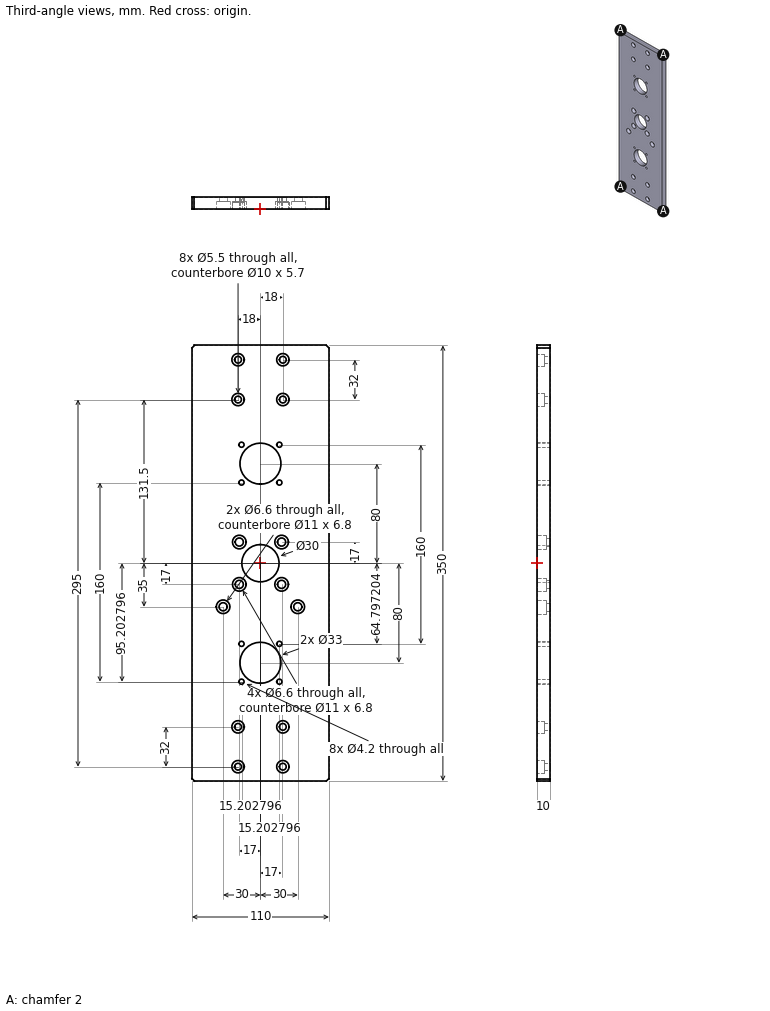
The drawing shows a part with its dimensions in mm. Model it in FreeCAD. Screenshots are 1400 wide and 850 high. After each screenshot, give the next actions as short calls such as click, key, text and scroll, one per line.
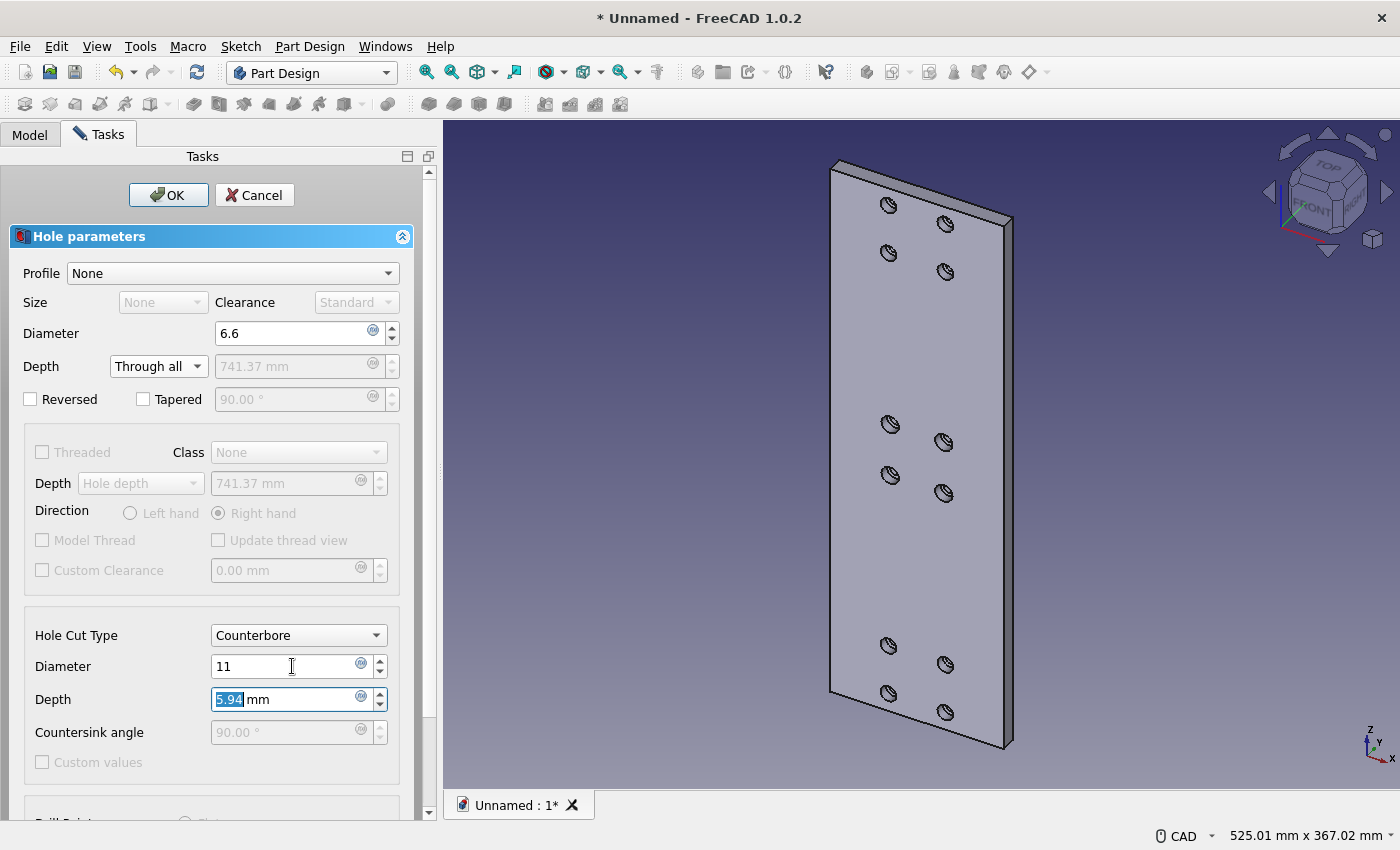
text(6.8)
key(Tab)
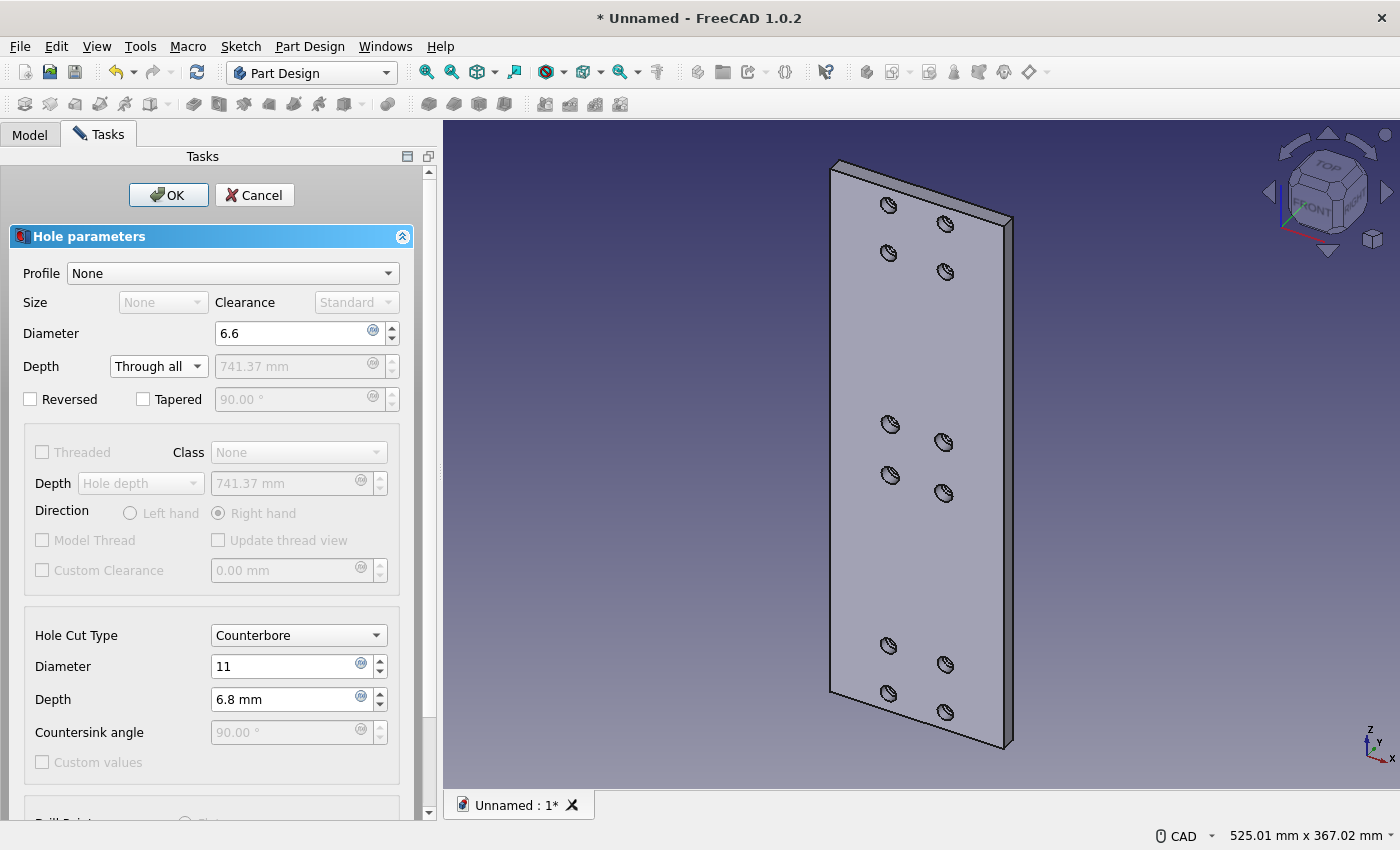
click(169, 195)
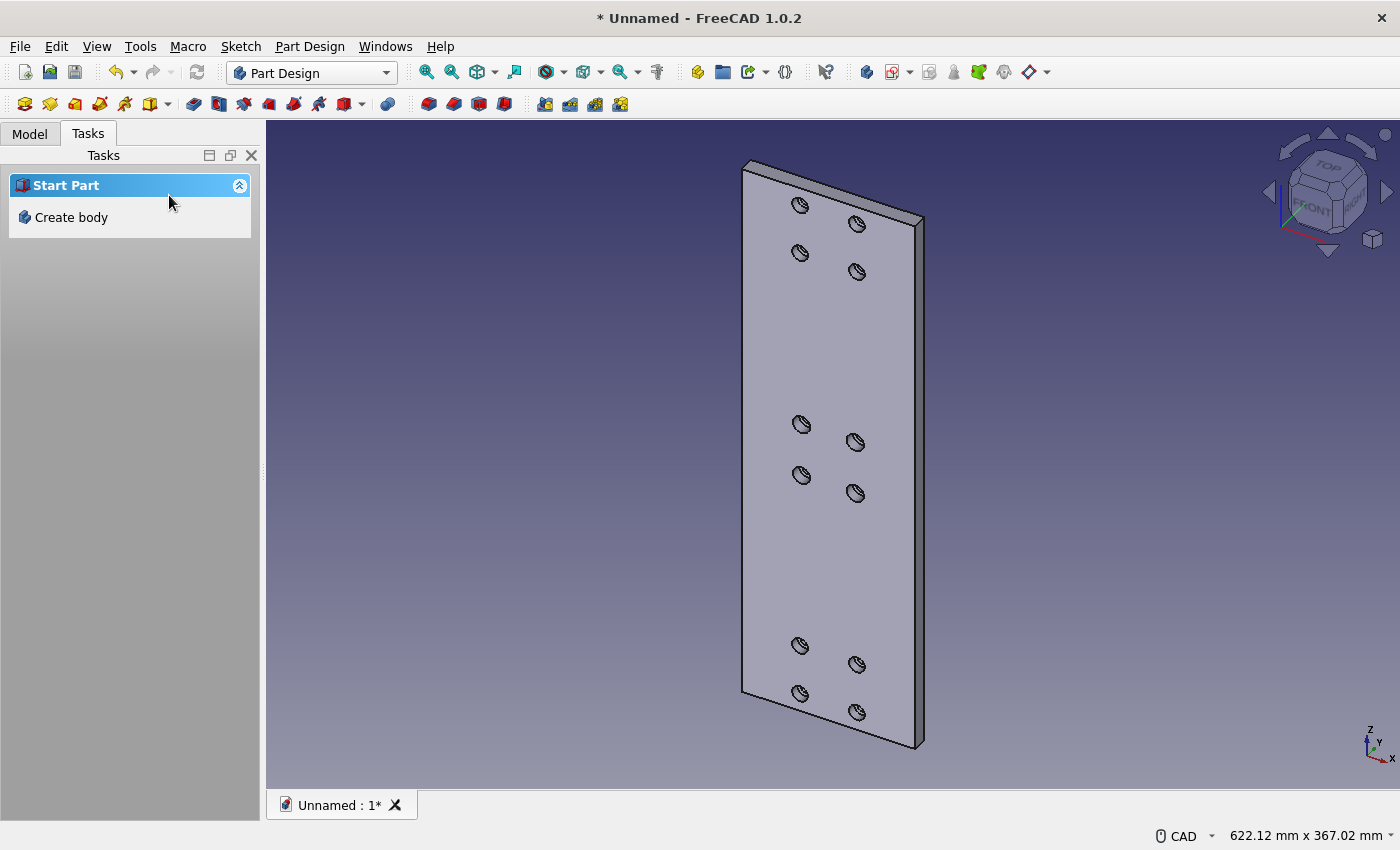
click(920, 221)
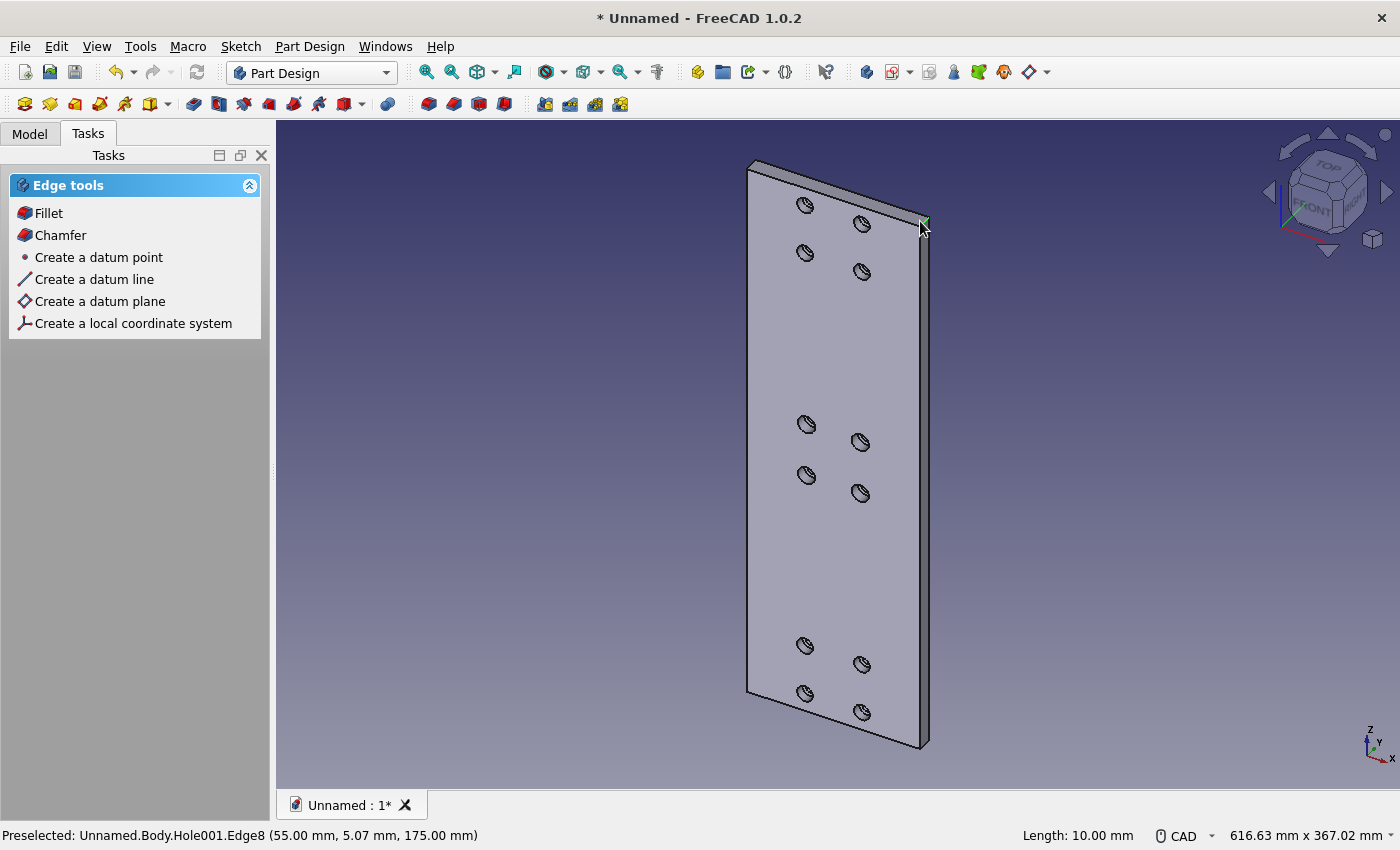
scroll(751, 163, up, 4)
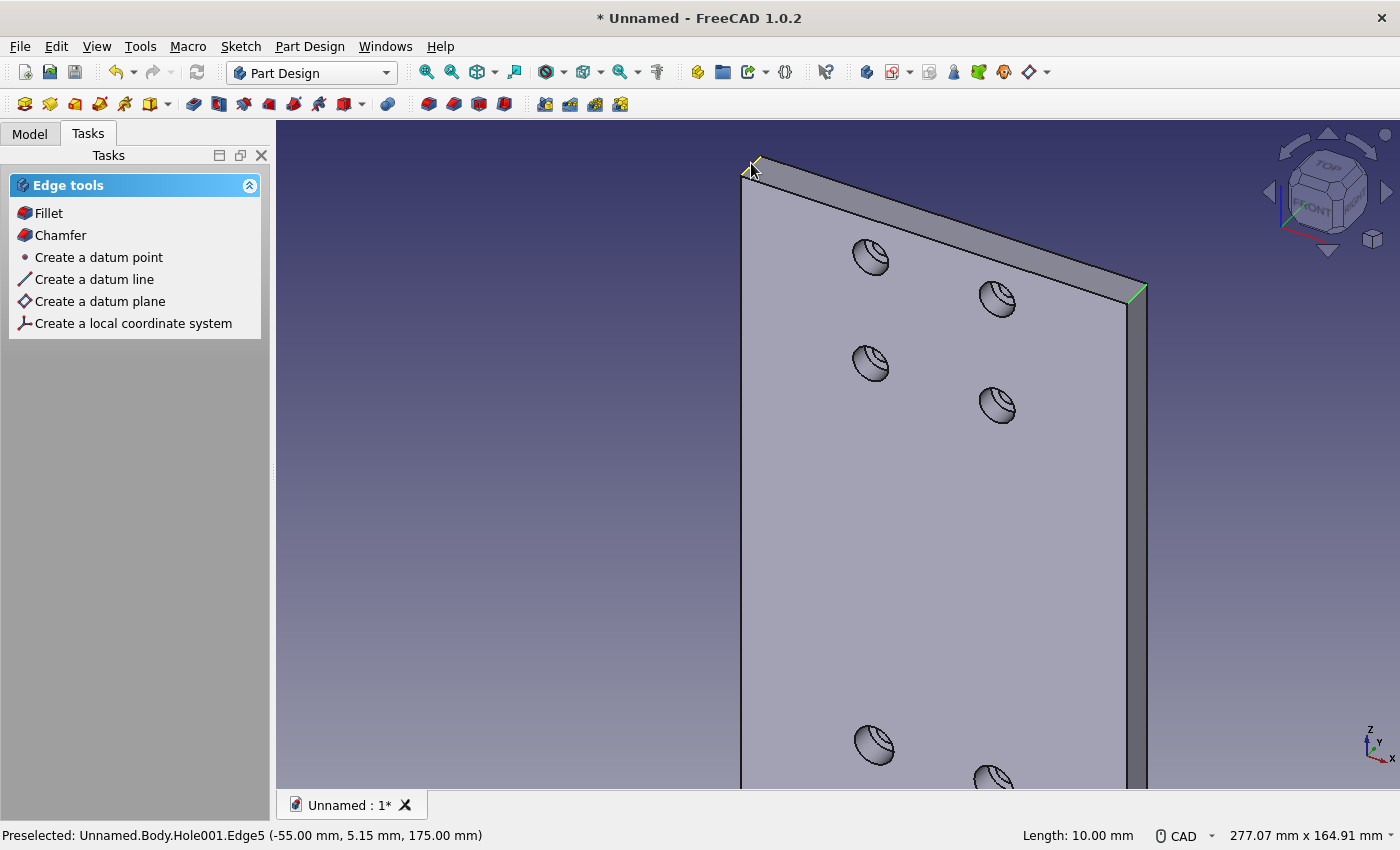
click(427, 72)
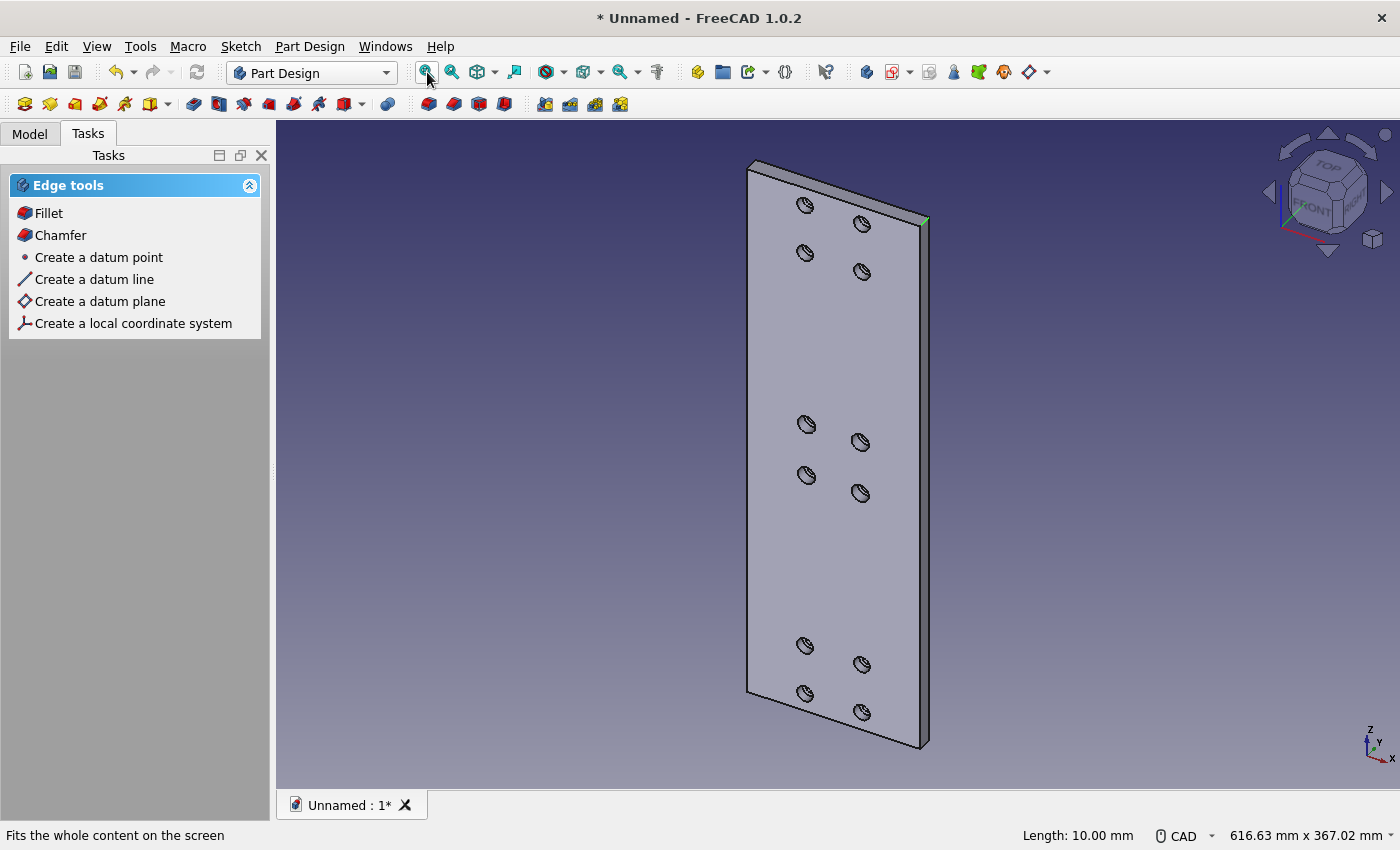
key(0)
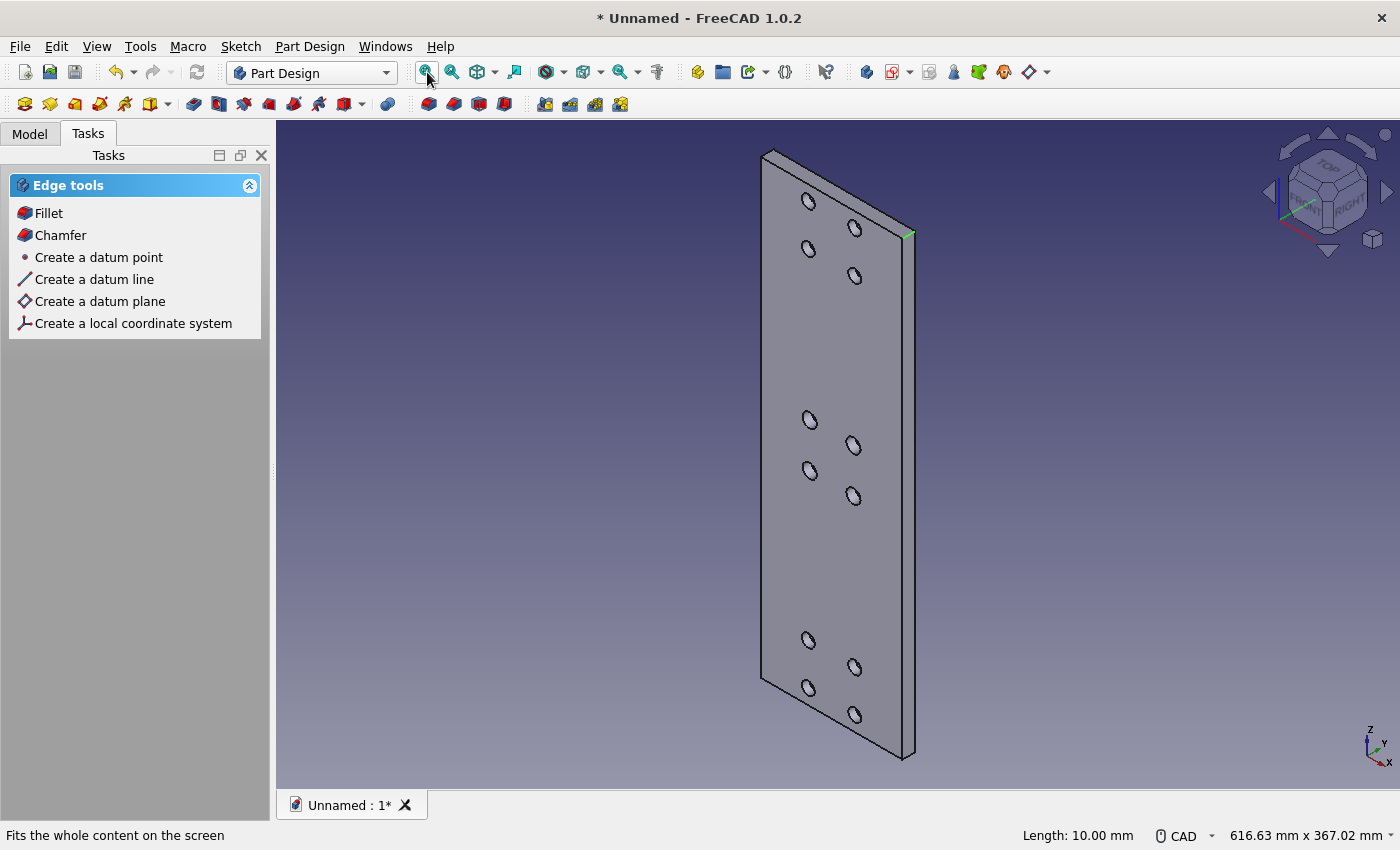
scroll(767, 152, up, 4)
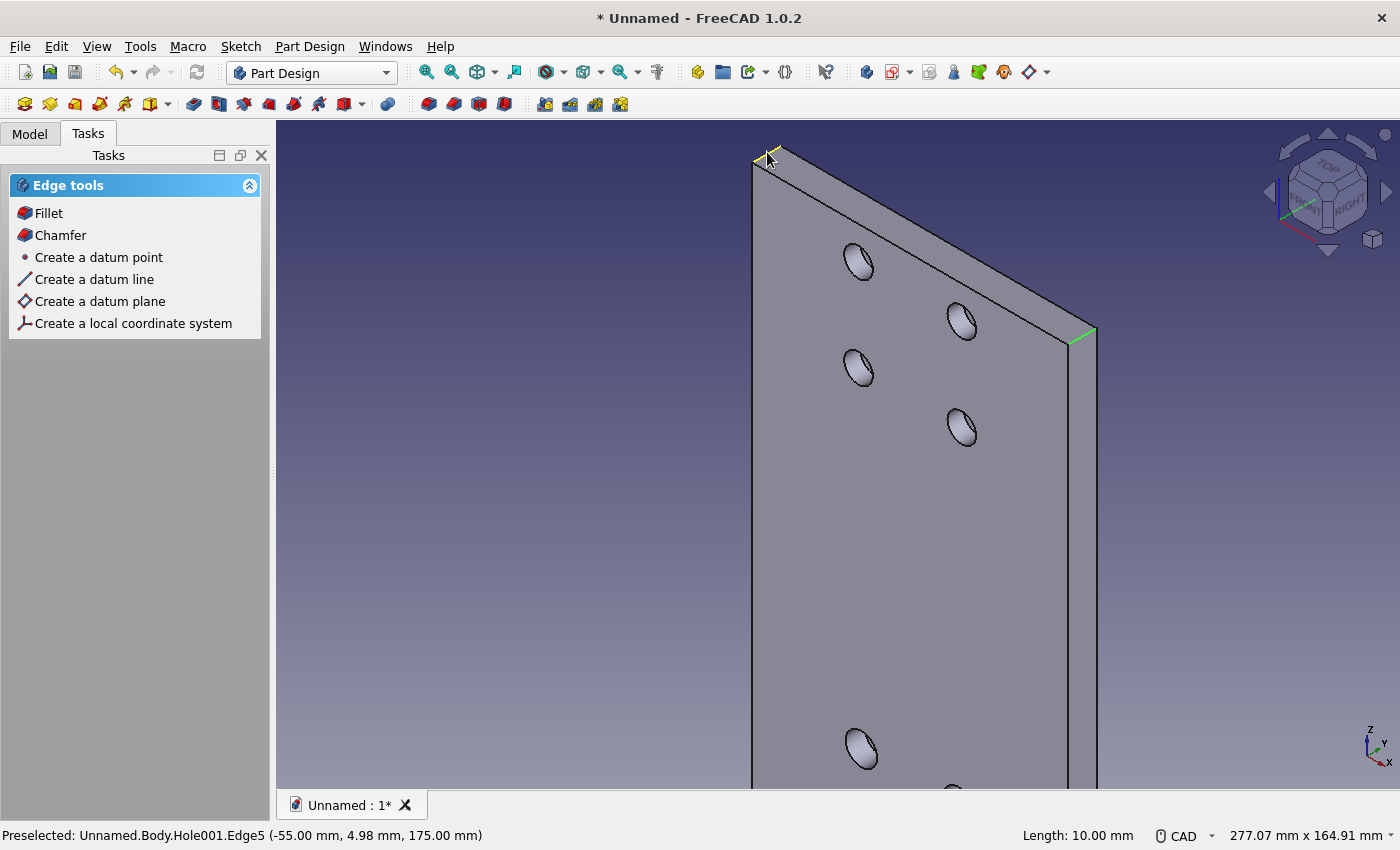
click(427, 72)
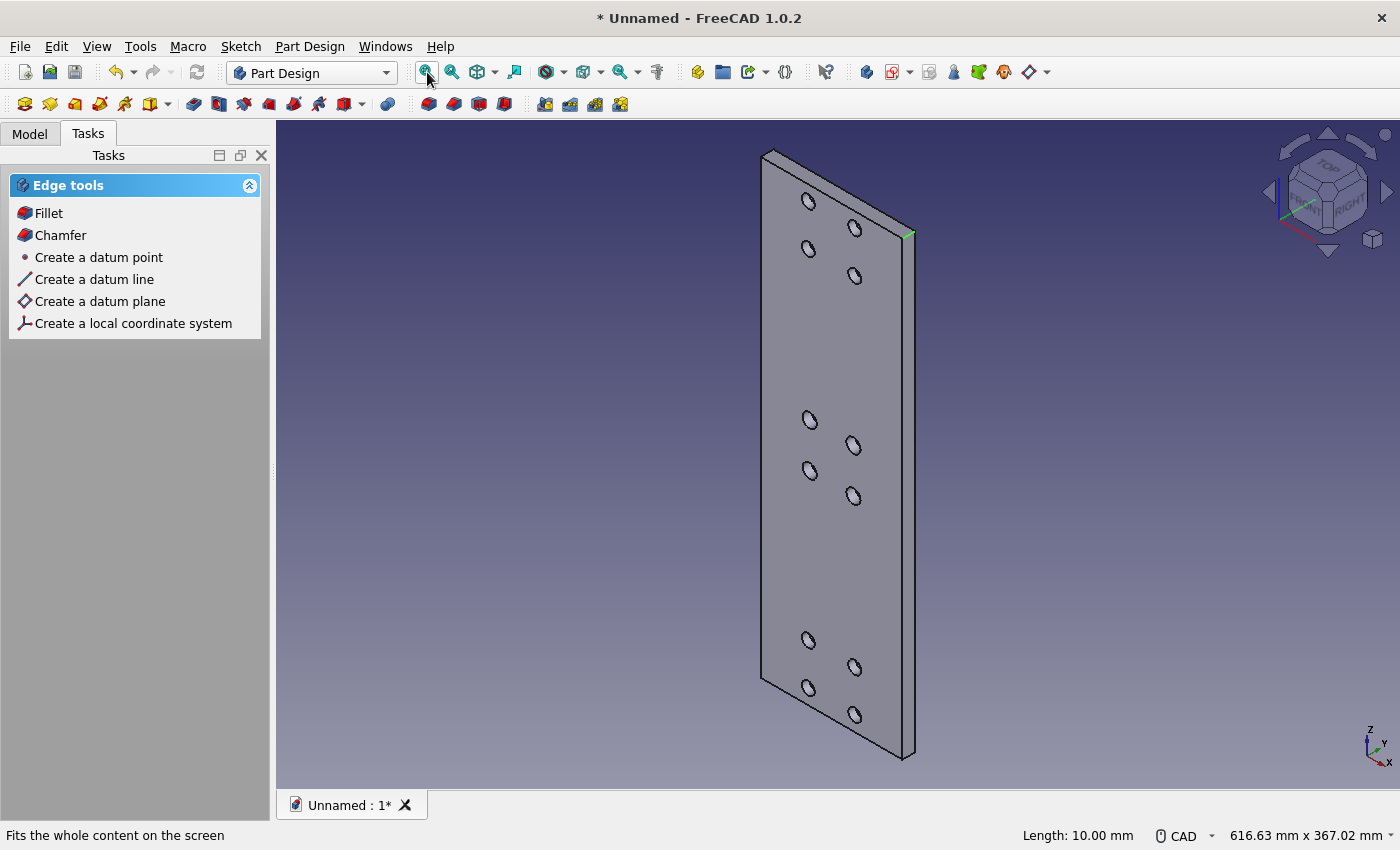
key(2)